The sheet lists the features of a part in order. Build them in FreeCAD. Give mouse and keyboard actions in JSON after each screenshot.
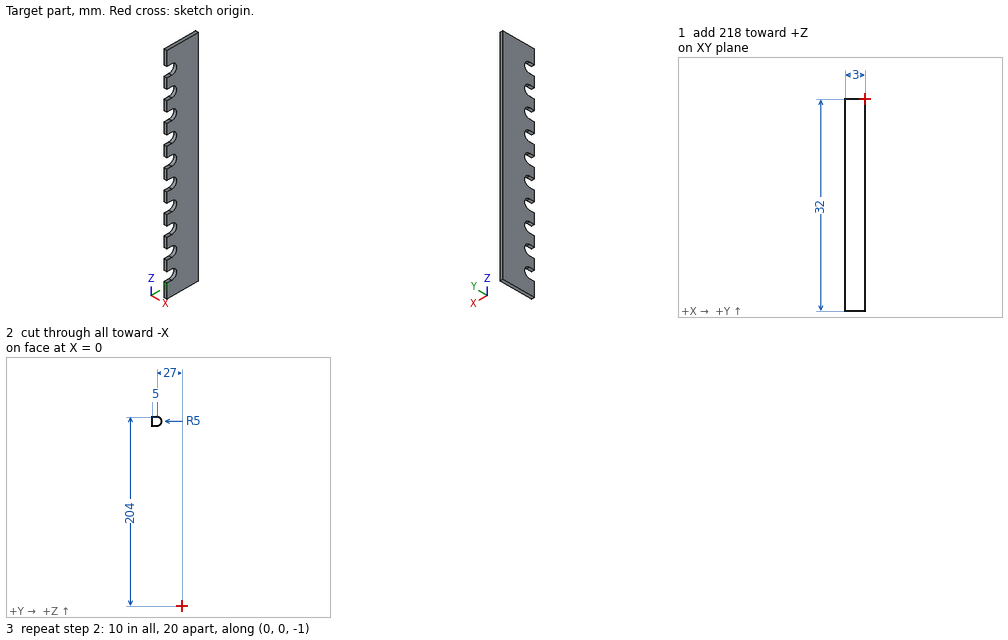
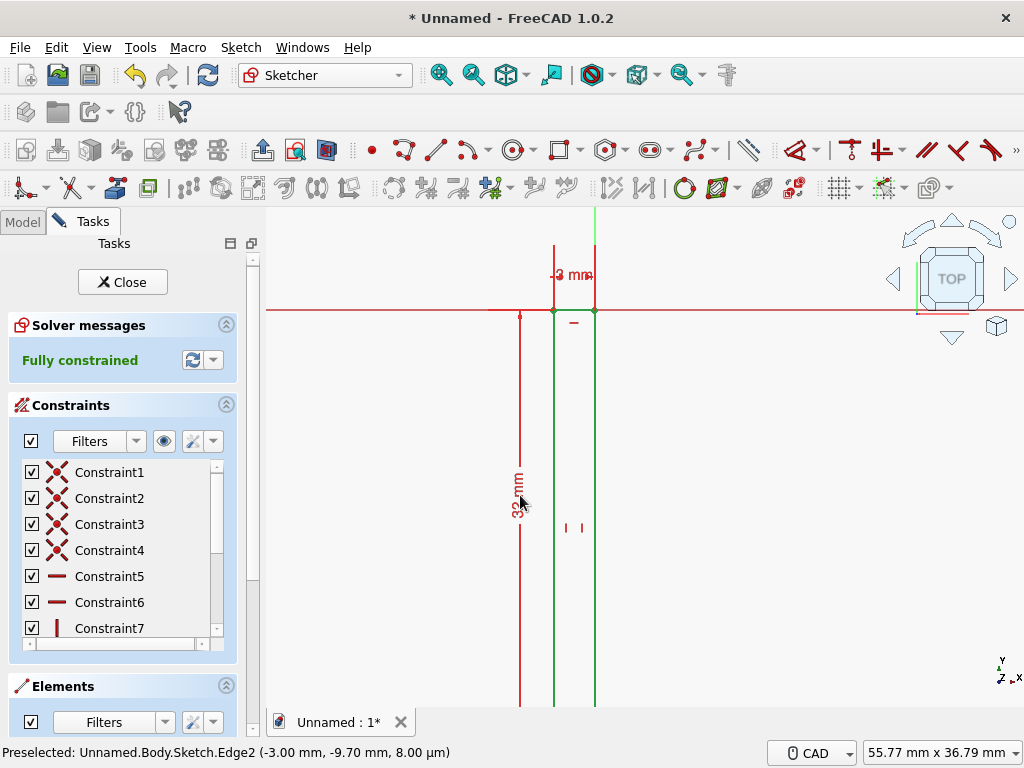
{"action": "left_click", "coordinate": [123, 282]}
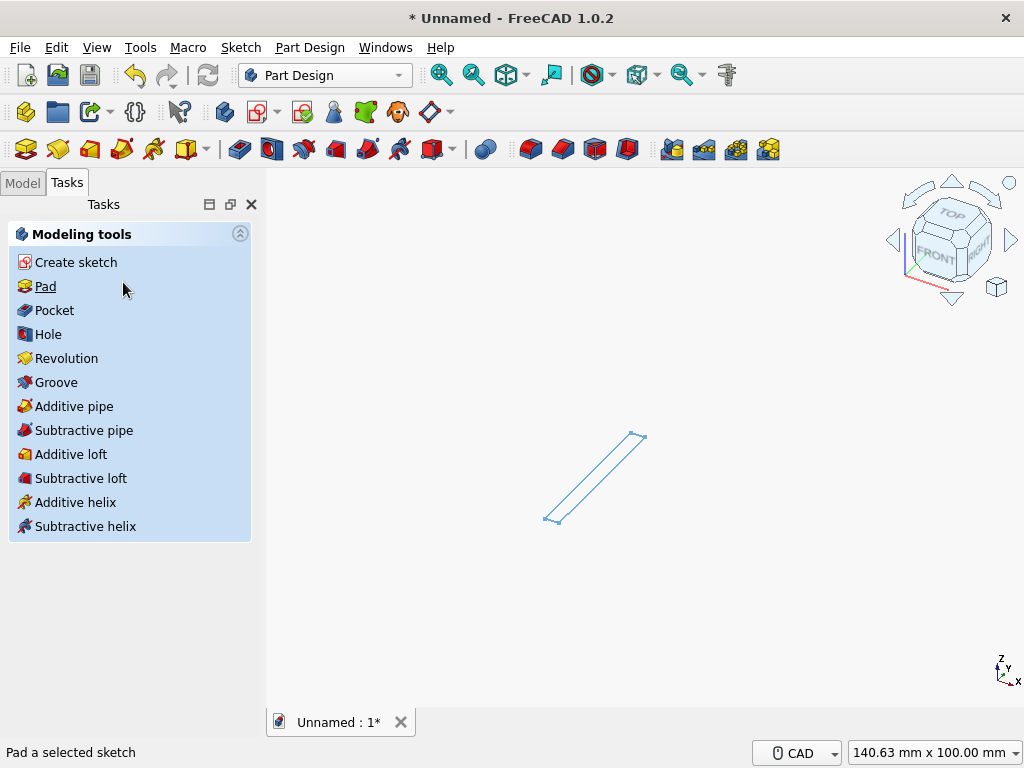
{"action": "left_click", "coordinate": [26, 150]}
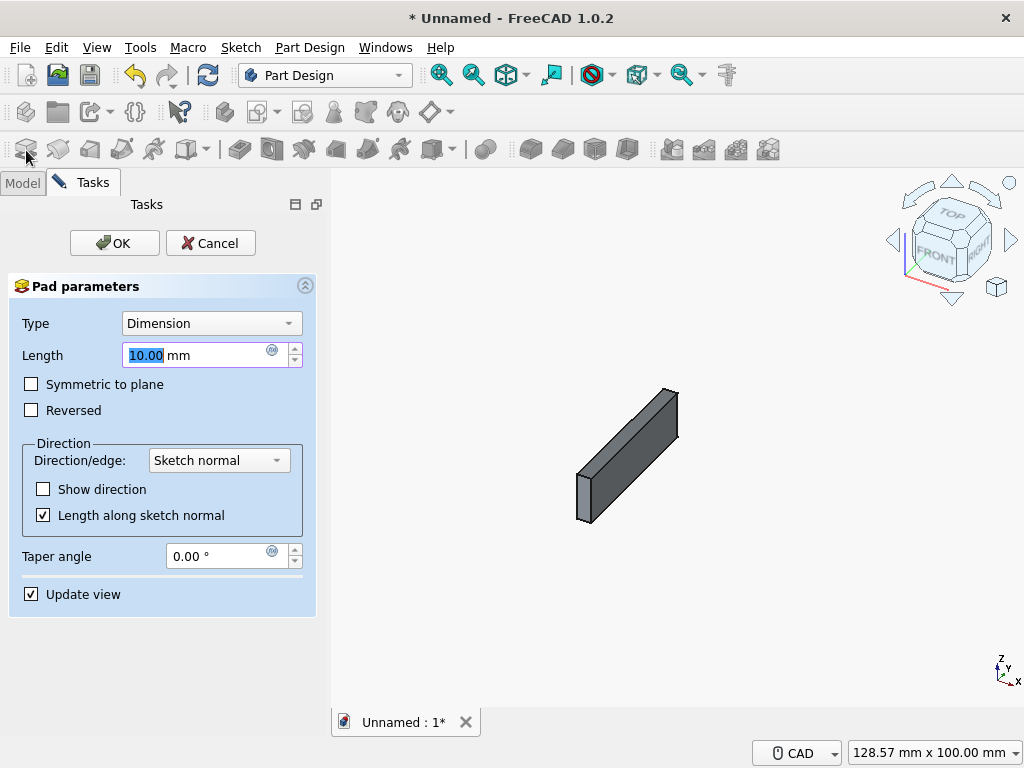
{"action": "type", "text": "218"}
{"action": "key", "text": "Tab"}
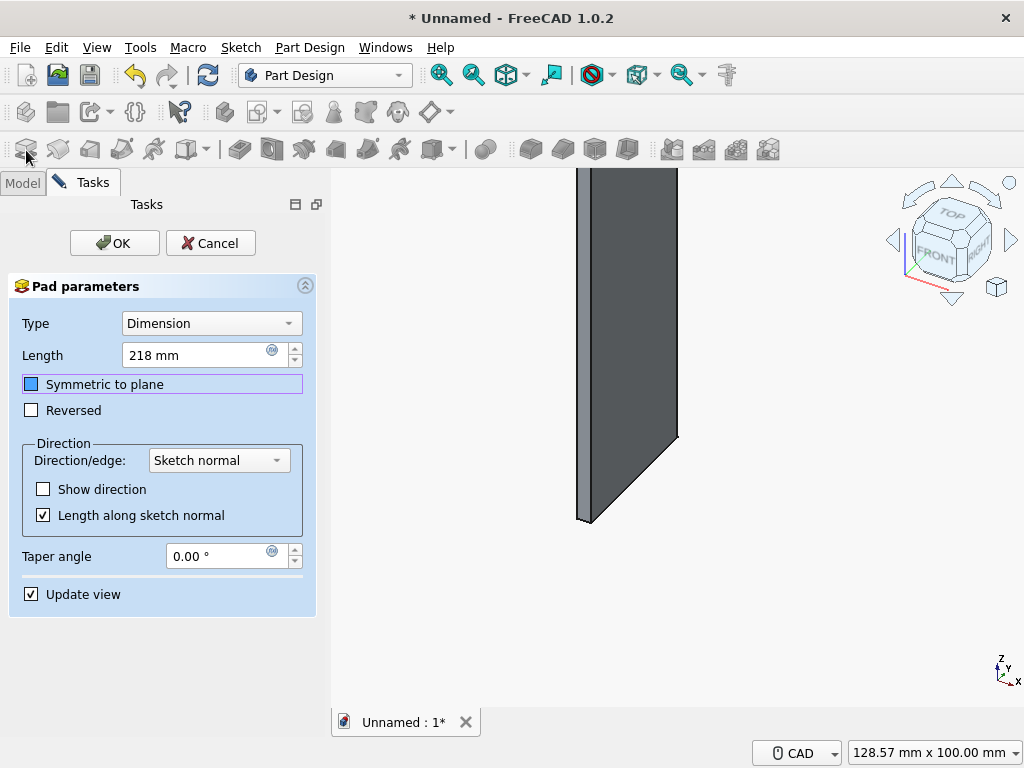
{"action": "left_click", "coordinate": [115, 243]}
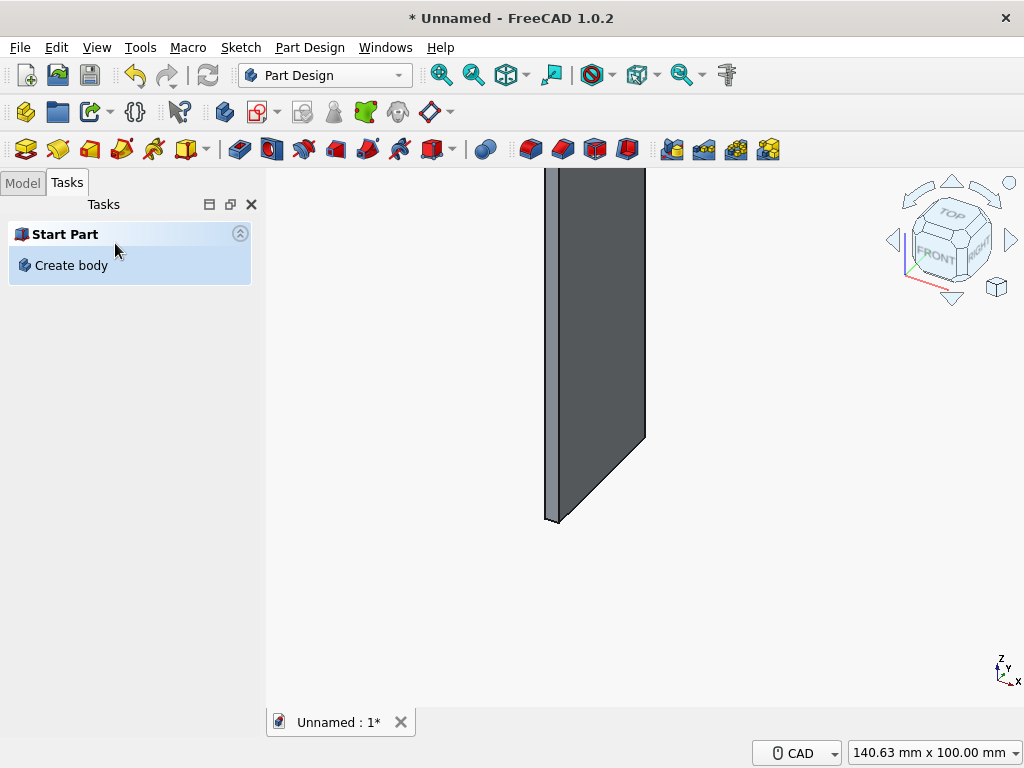
{"action": "left_click", "coordinate": [442, 76]}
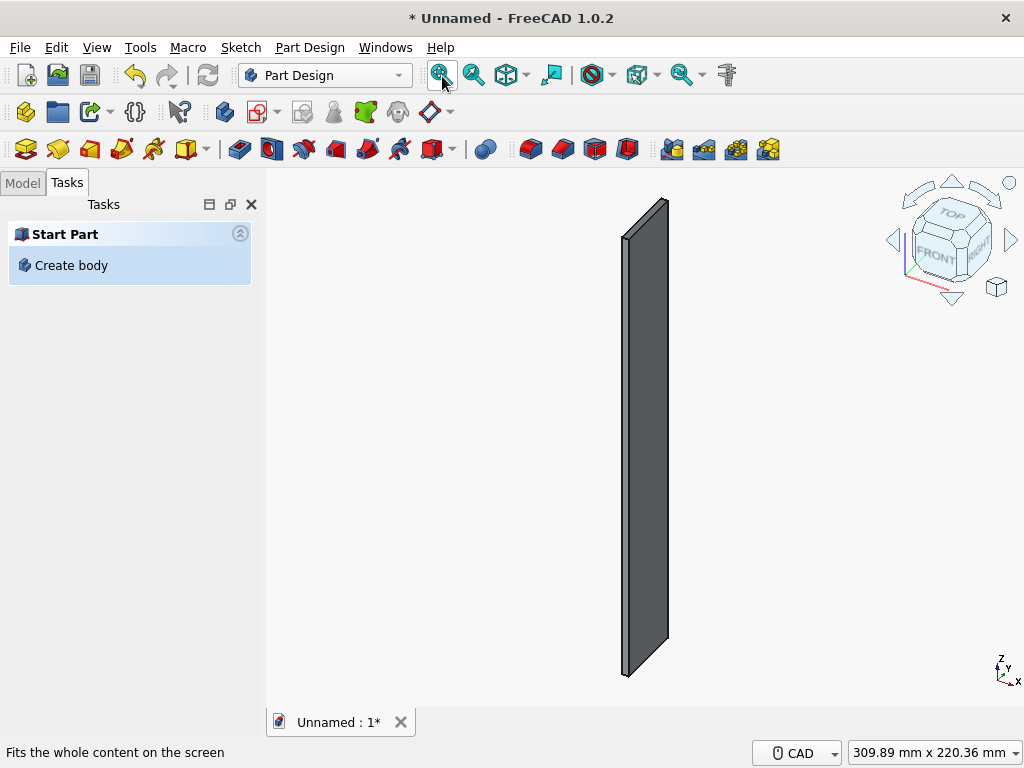
{"action": "left_click", "coordinate": [648, 313]}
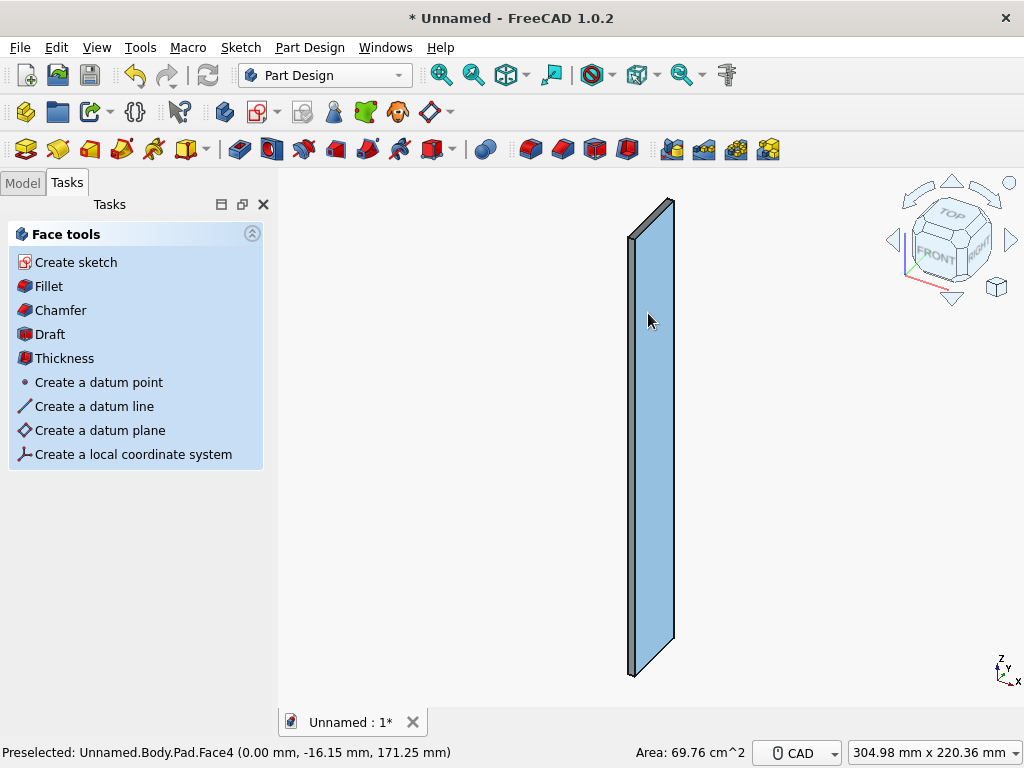
{"action": "left_click", "coordinate": [258, 112]}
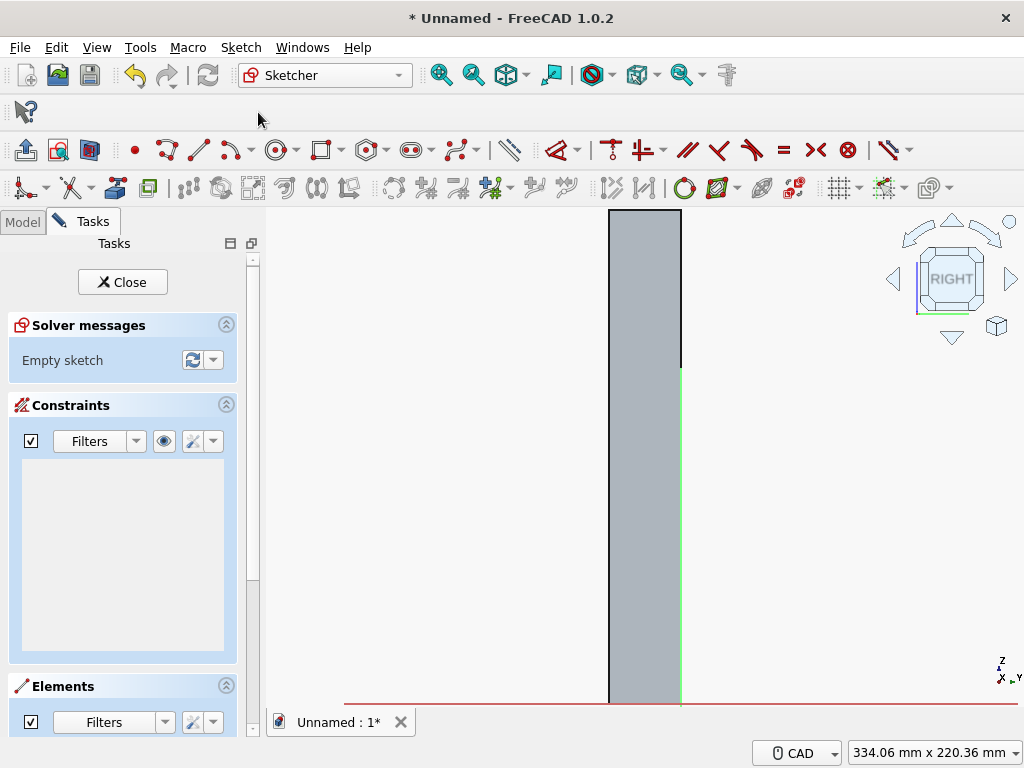
{"action": "scroll", "coordinate": [624, 236], "scroll_direction": "up", "scroll_amount": 13}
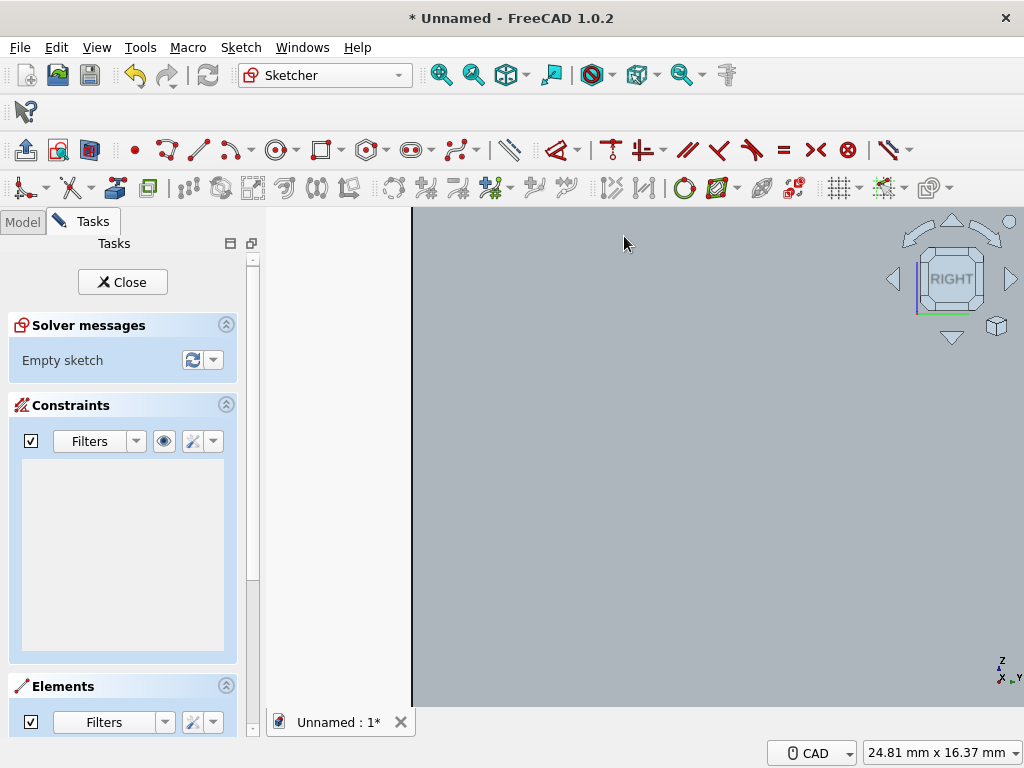
{"action": "left_click", "coordinate": [168, 150]}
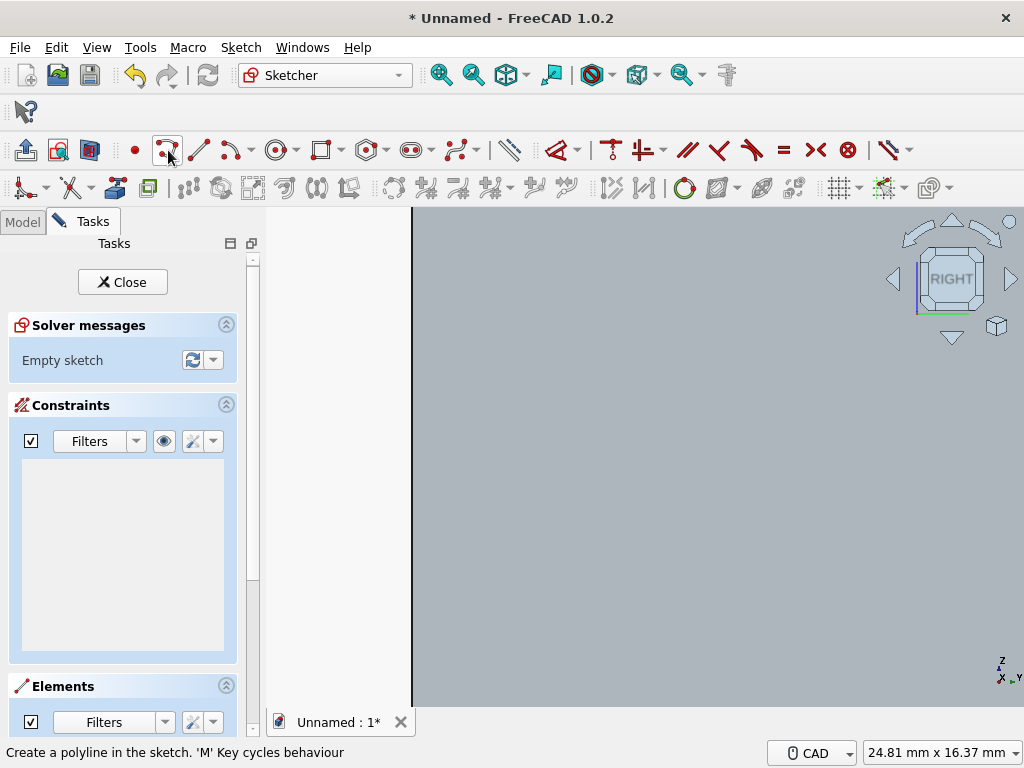
{"action": "left_click", "coordinate": [565, 309]}
{"action": "left_click", "coordinate": [412, 309]}
{"action": "left_click", "coordinate": [412, 614]}
{"action": "left_click", "coordinate": [565, 614]}
{"action": "right_click", "coordinate": [565, 614]}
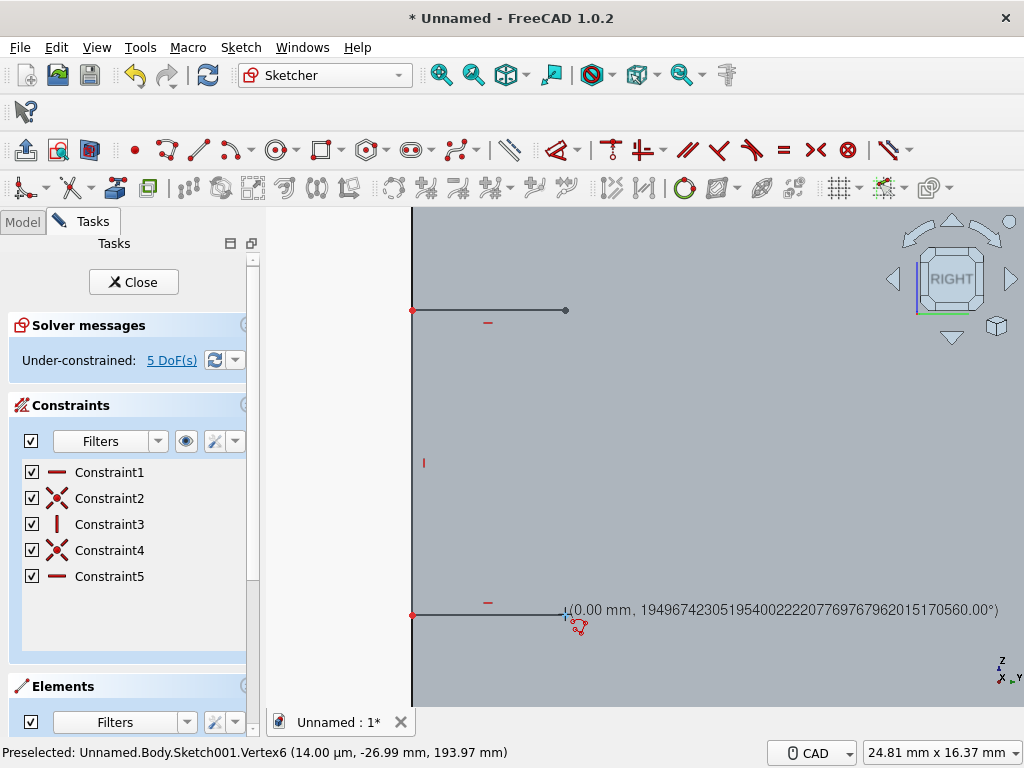
{"action": "left_click", "coordinate": [254, 150]}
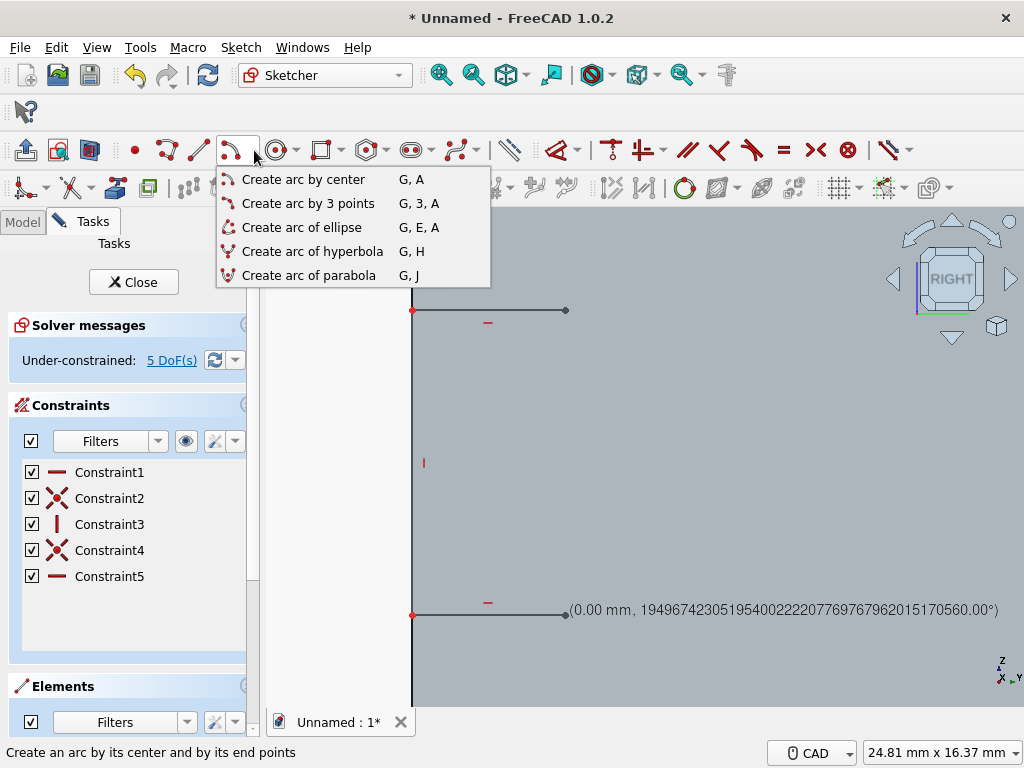
{"action": "left_click", "coordinate": [354, 203]}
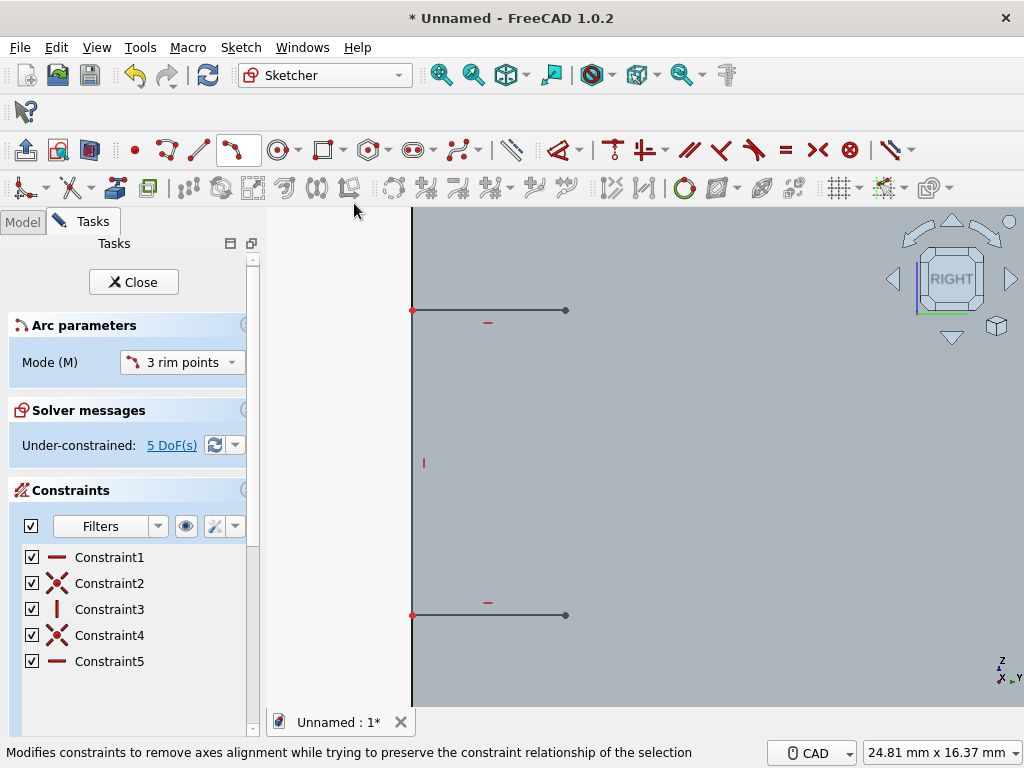
{"action": "left_click", "coordinate": [565, 615]}
{"action": "left_click", "coordinate": [565, 310]}
{"action": "left_click", "coordinate": [718, 461]}
{"action": "key", "text": "Escape"}